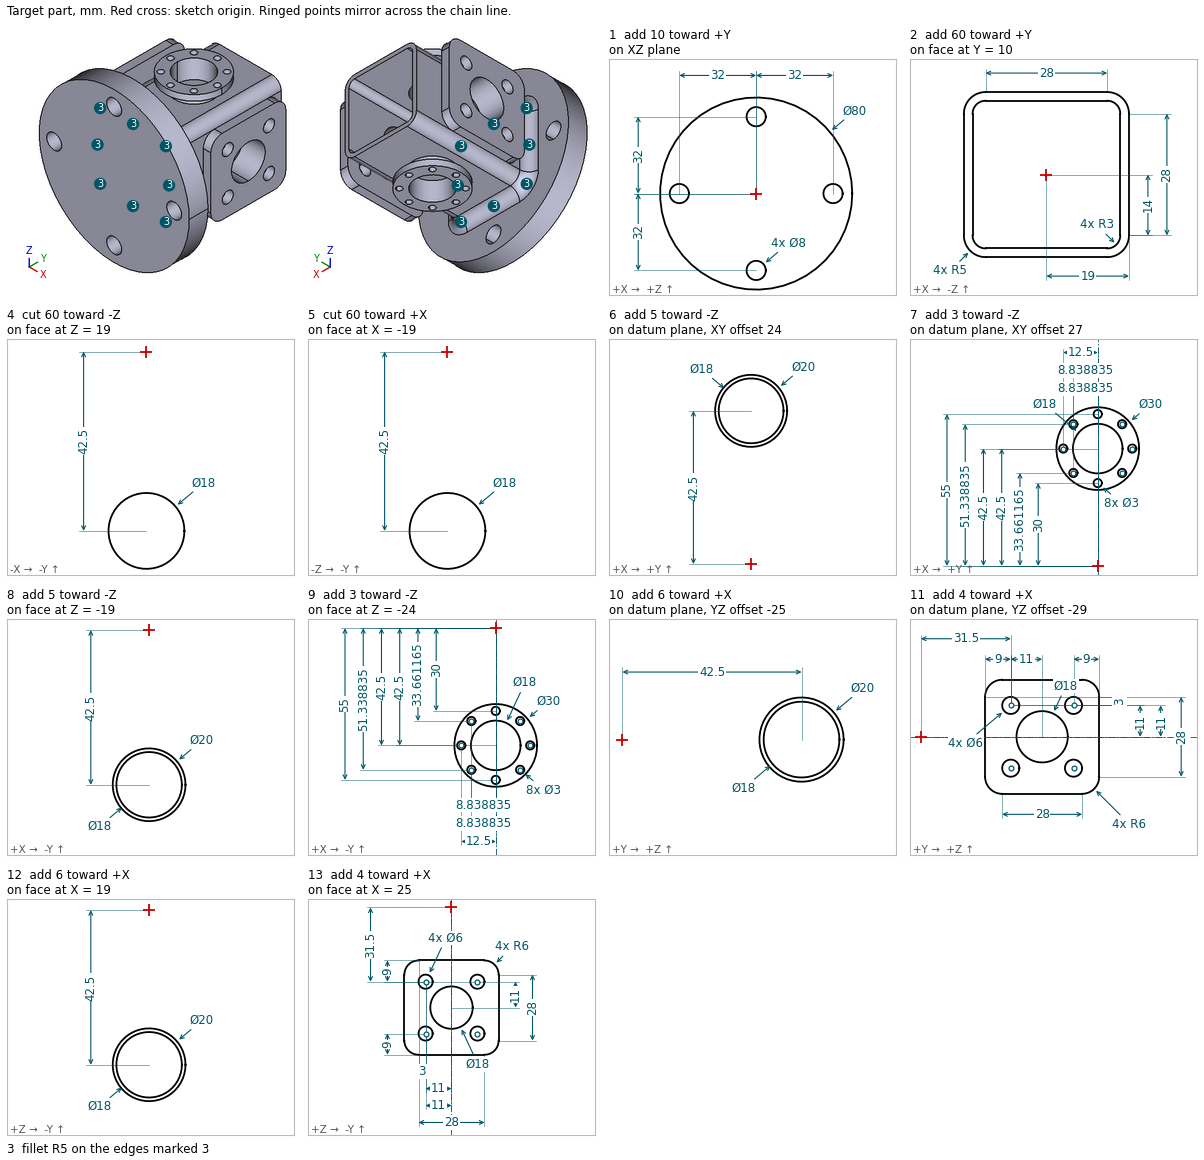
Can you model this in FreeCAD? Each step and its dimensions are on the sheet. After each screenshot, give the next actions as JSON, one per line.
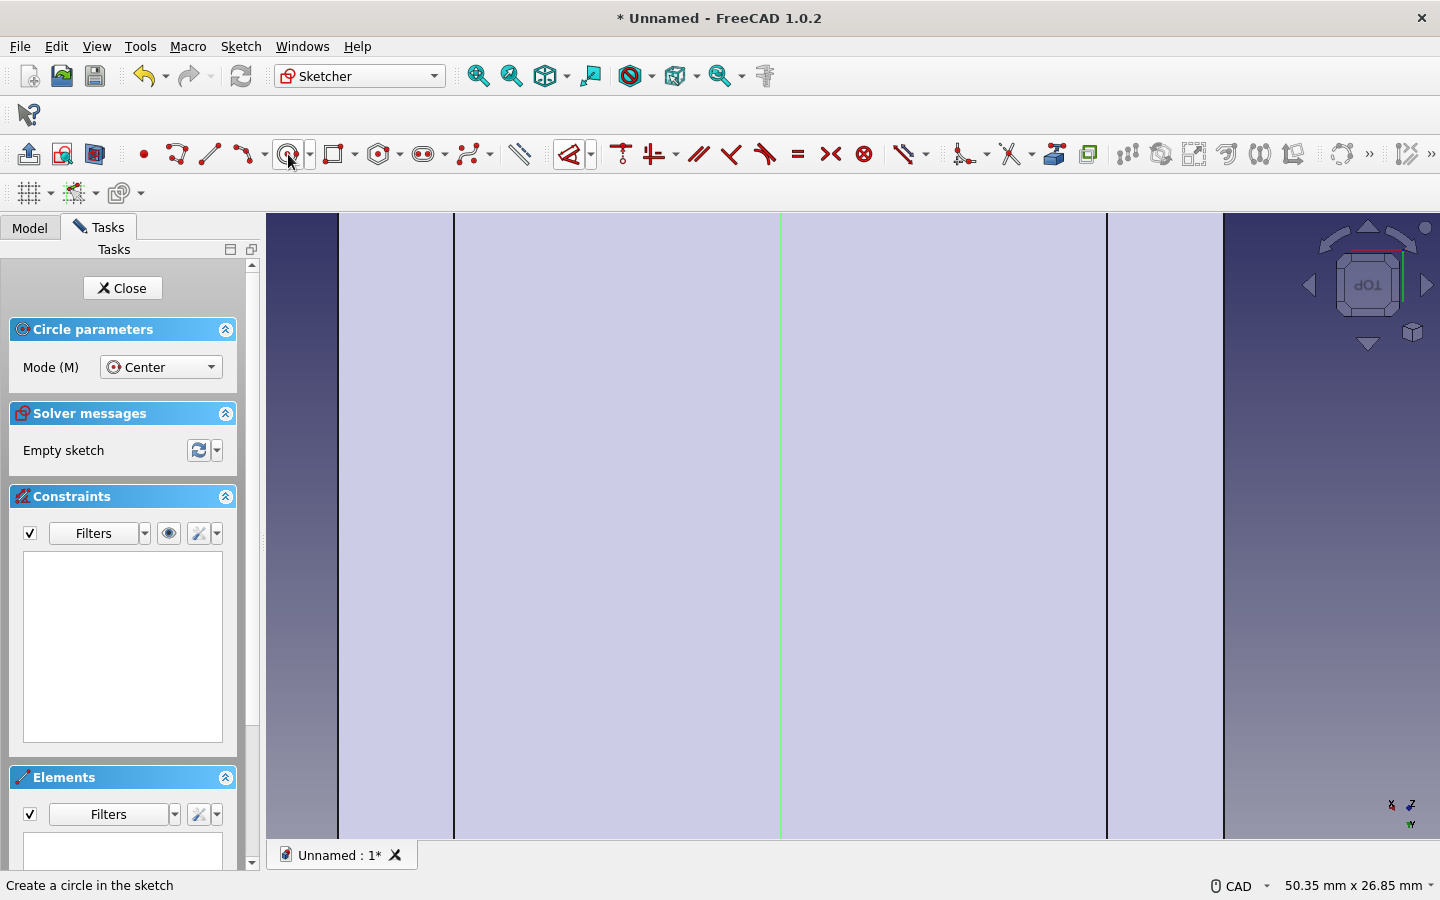
{"action": "left_click", "coordinate": [781, 525]}
{"action": "mouse_move", "coordinate": [929, 376]}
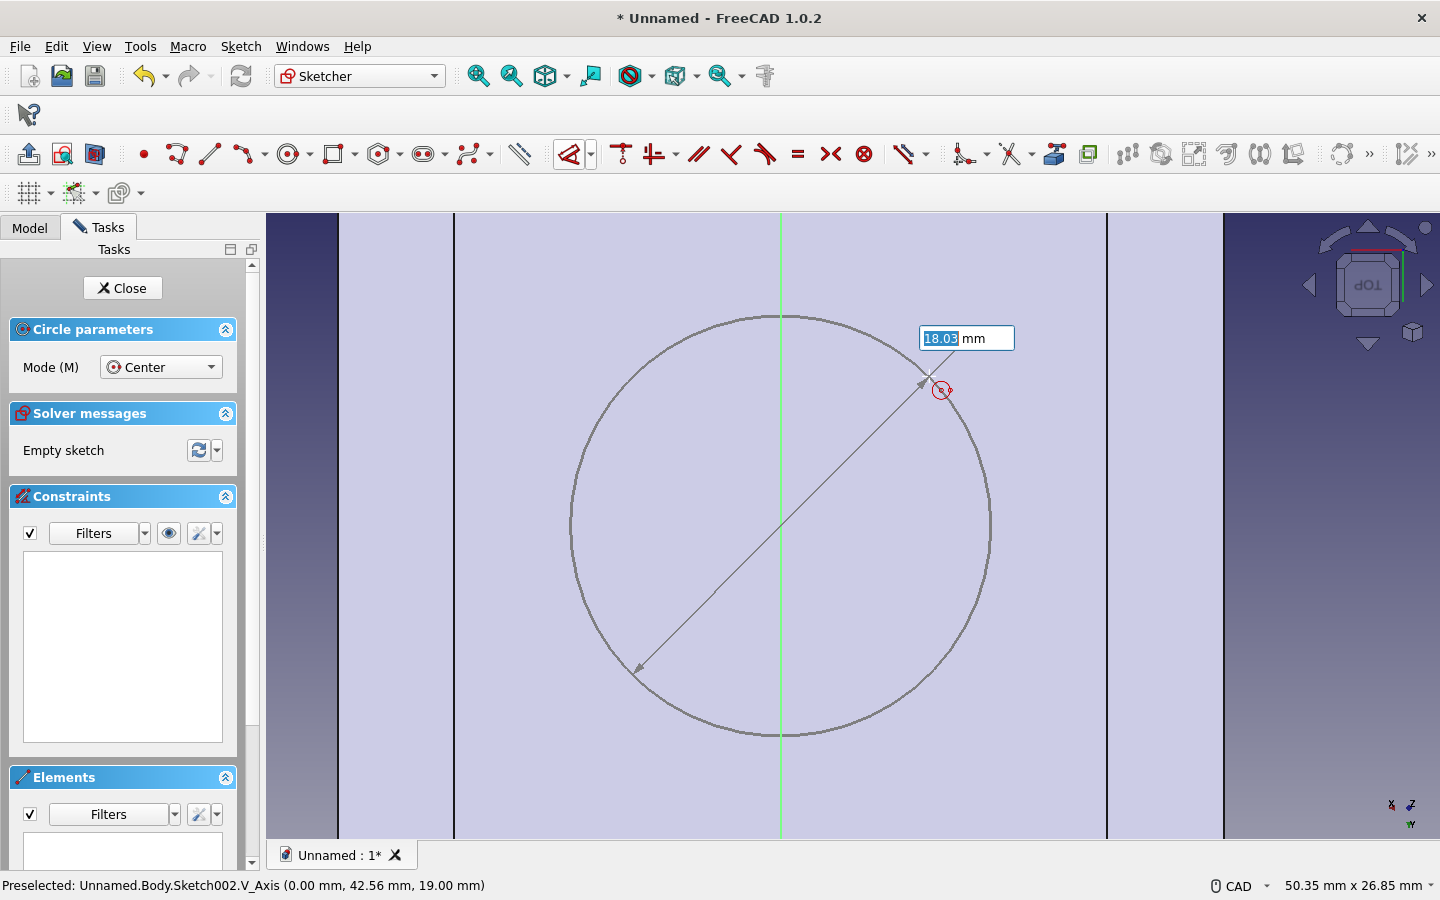
{"action": "type", "text": "18"}
{"action": "key", "text": "Return"}
{"action": "key", "text": "Escape"}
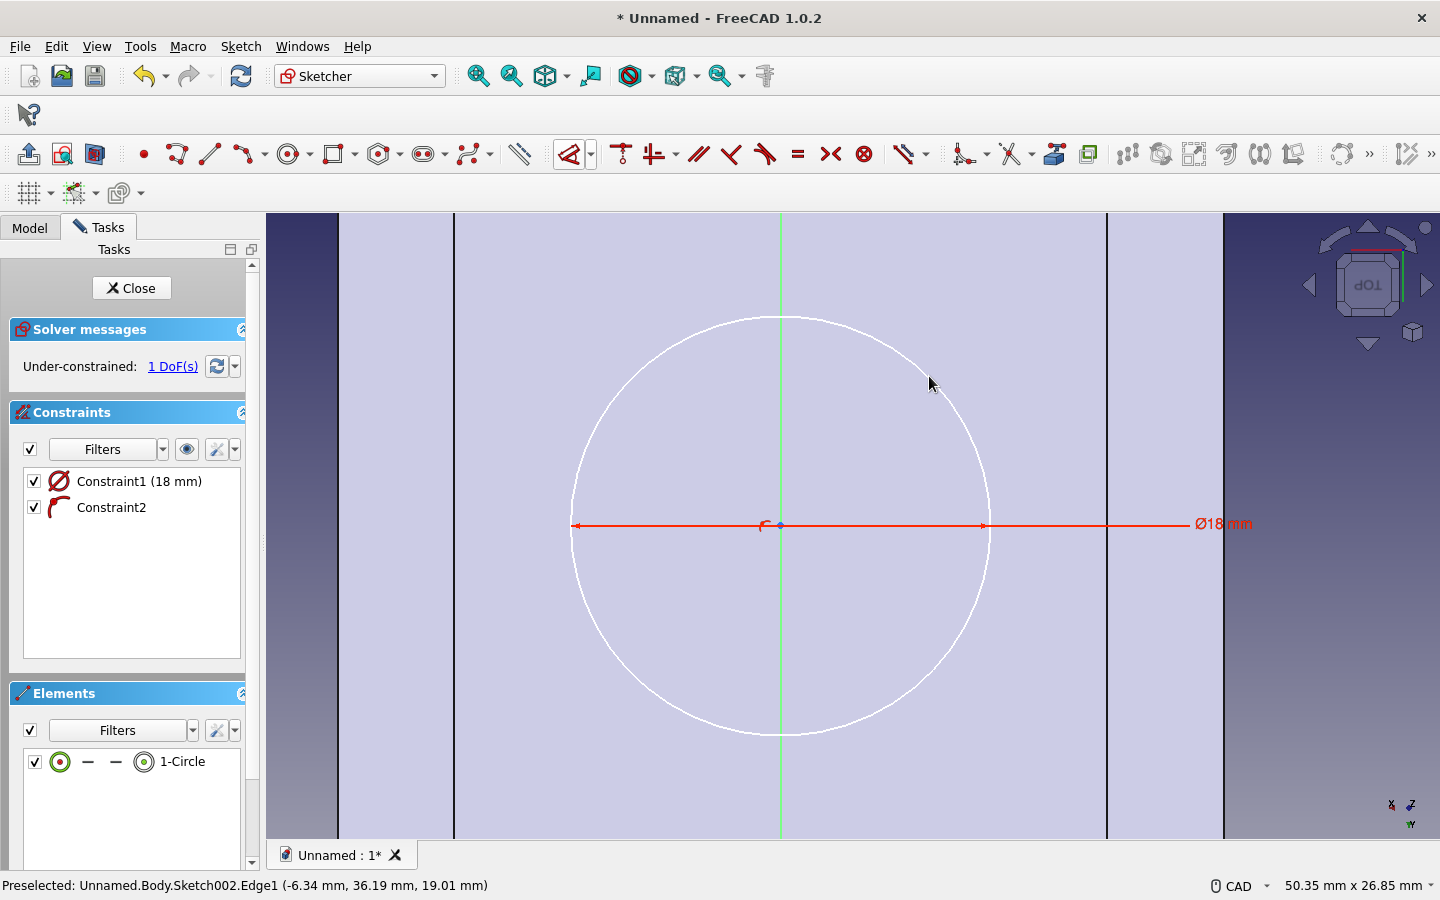
{"action": "left_click", "coordinate": [781, 526]}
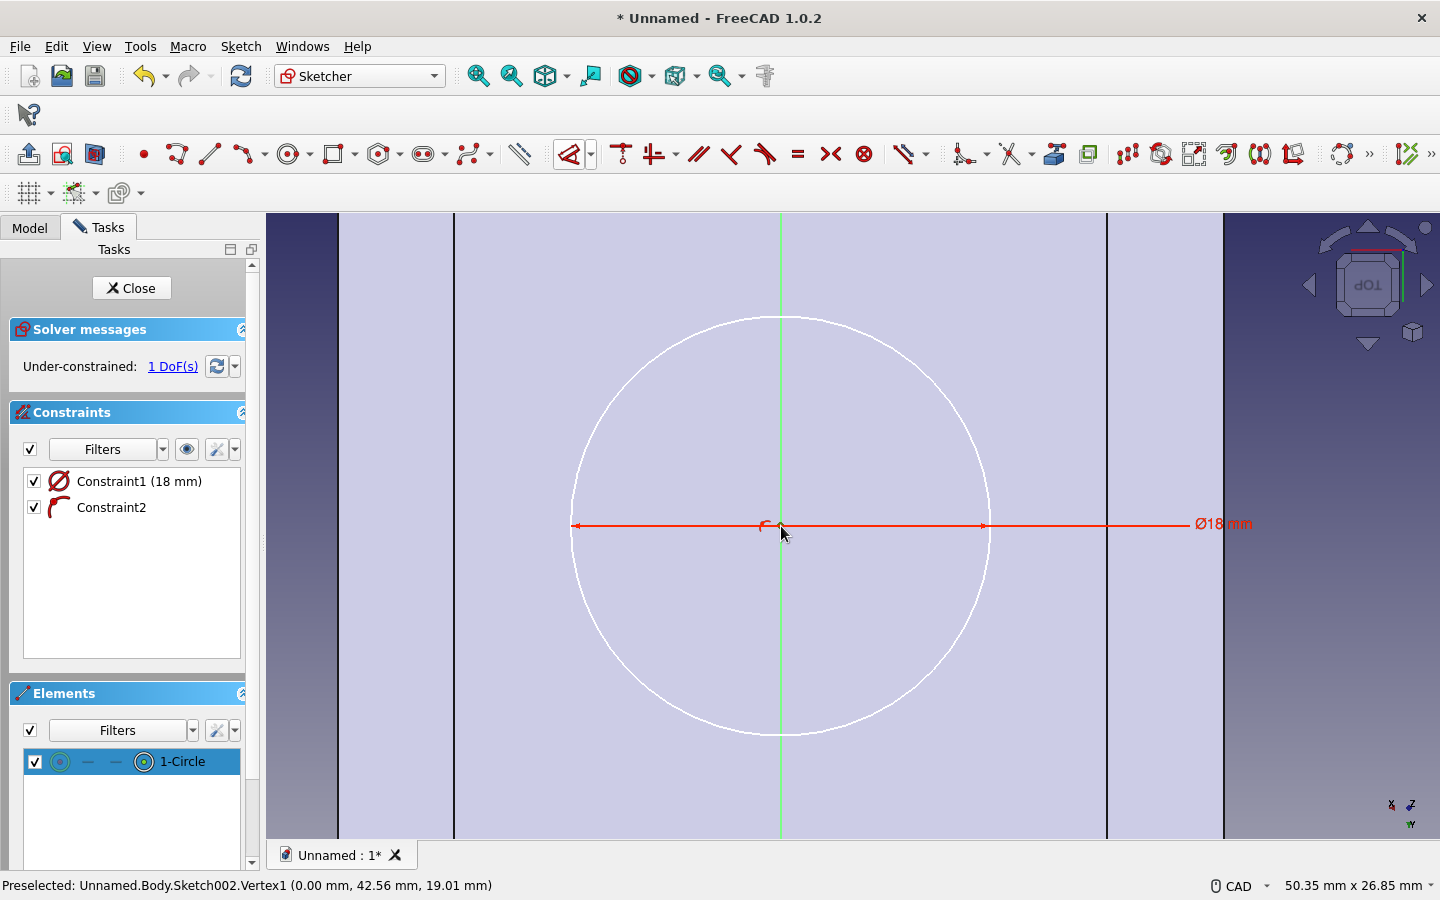
{"action": "key", "text": "i"}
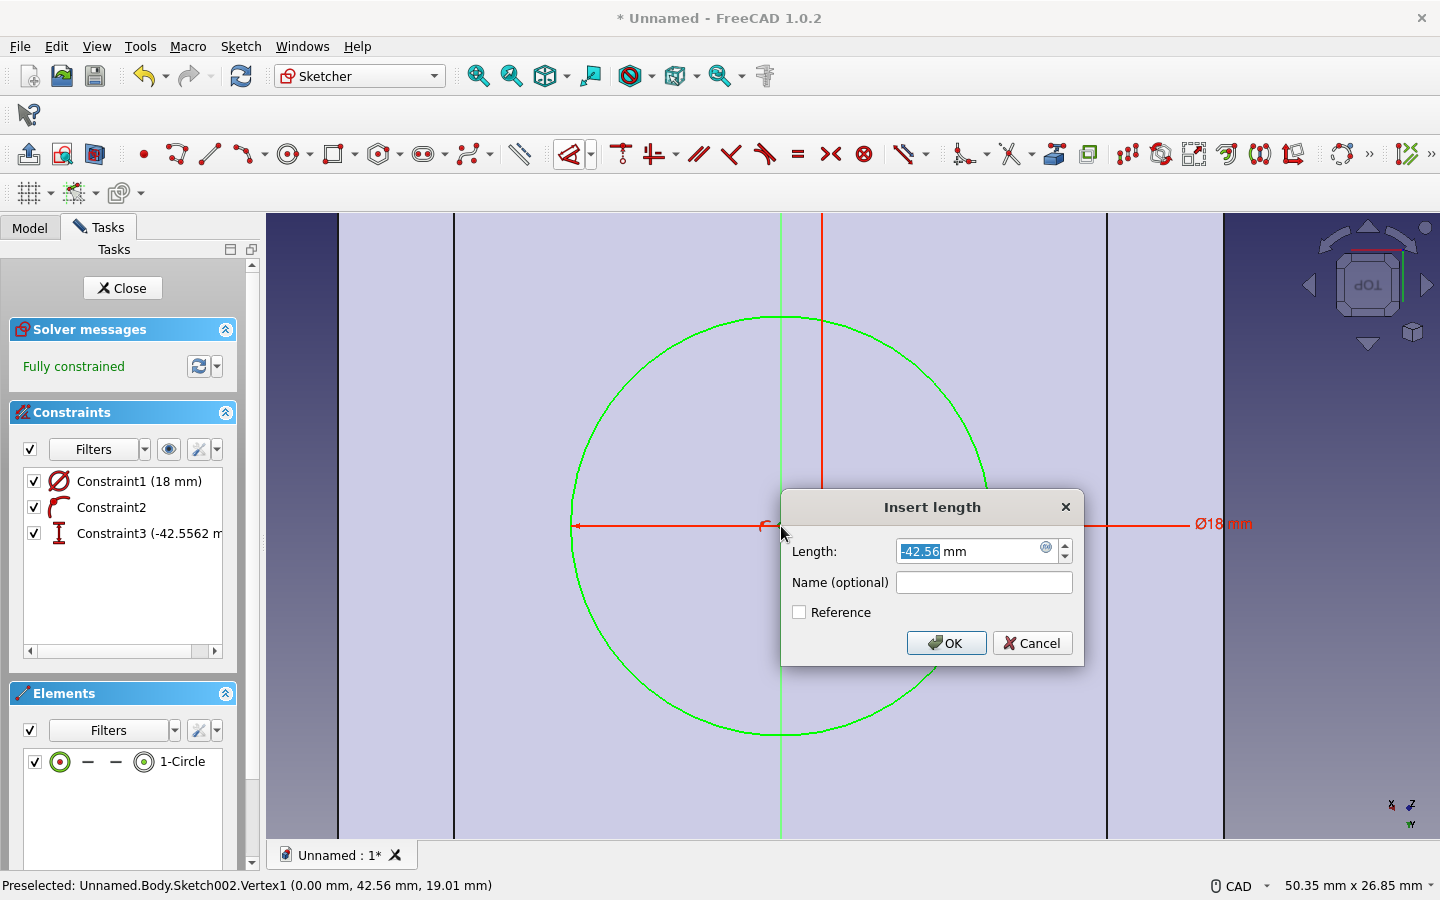
{"action": "type", "text": "-42.5"}
{"action": "key", "text": "Return"}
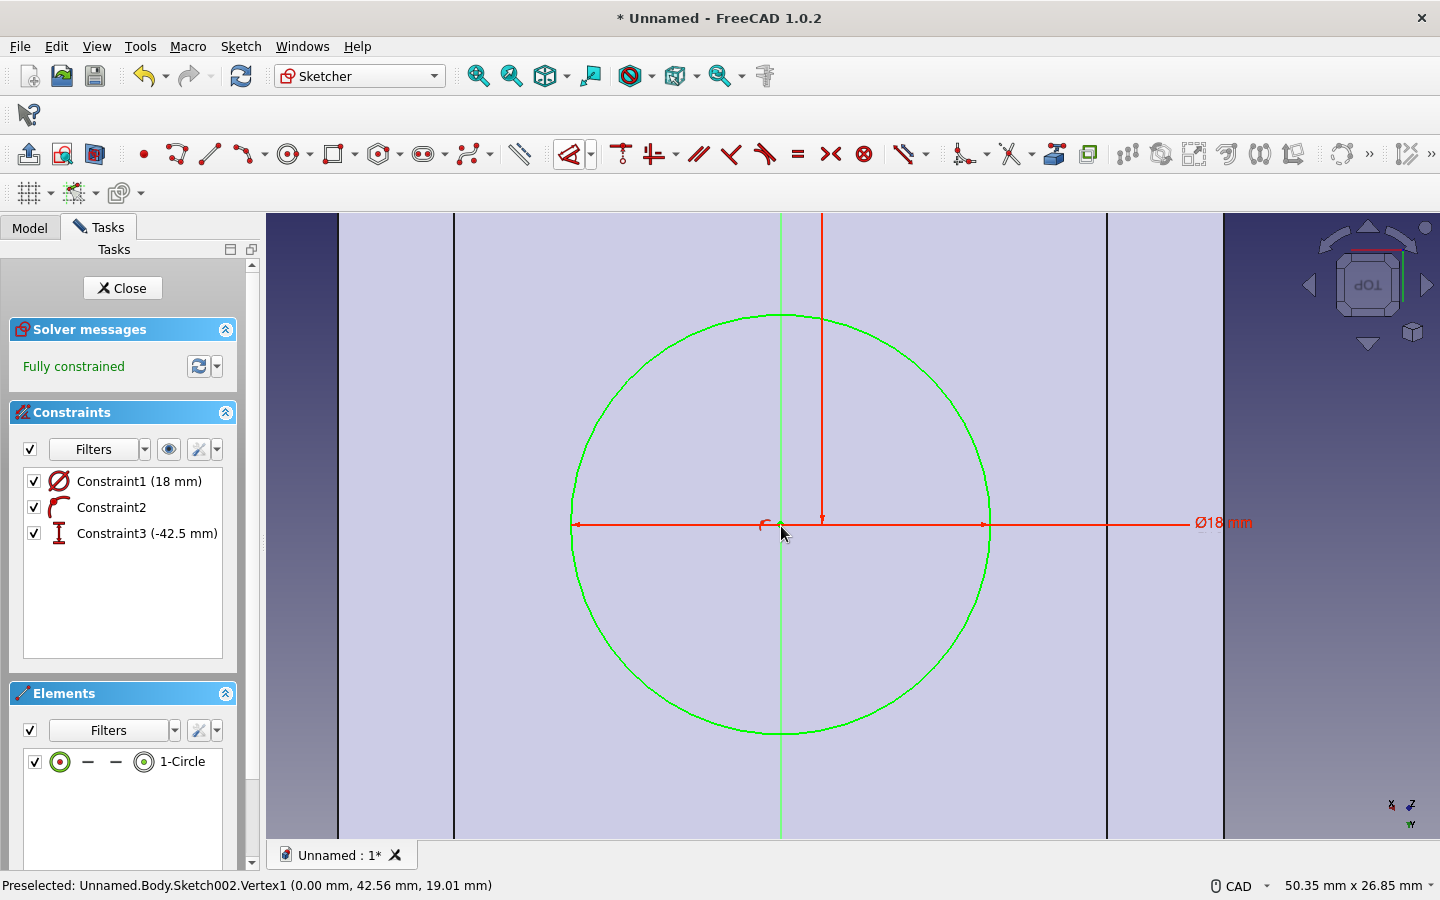
{"action": "left_click", "coordinate": [123, 288]}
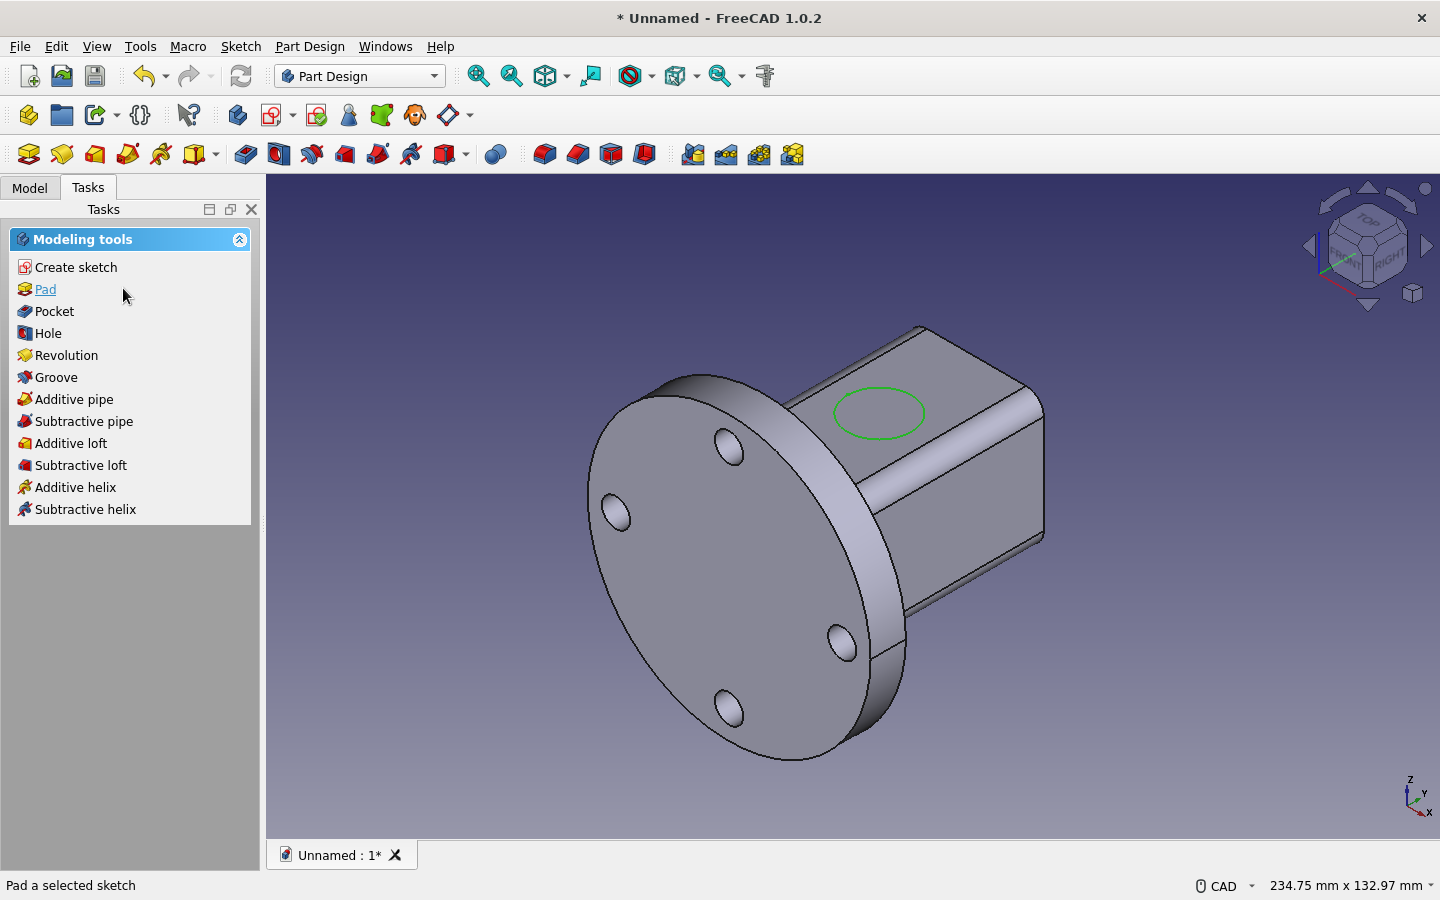
{"action": "left_click", "coordinate": [246, 154]}